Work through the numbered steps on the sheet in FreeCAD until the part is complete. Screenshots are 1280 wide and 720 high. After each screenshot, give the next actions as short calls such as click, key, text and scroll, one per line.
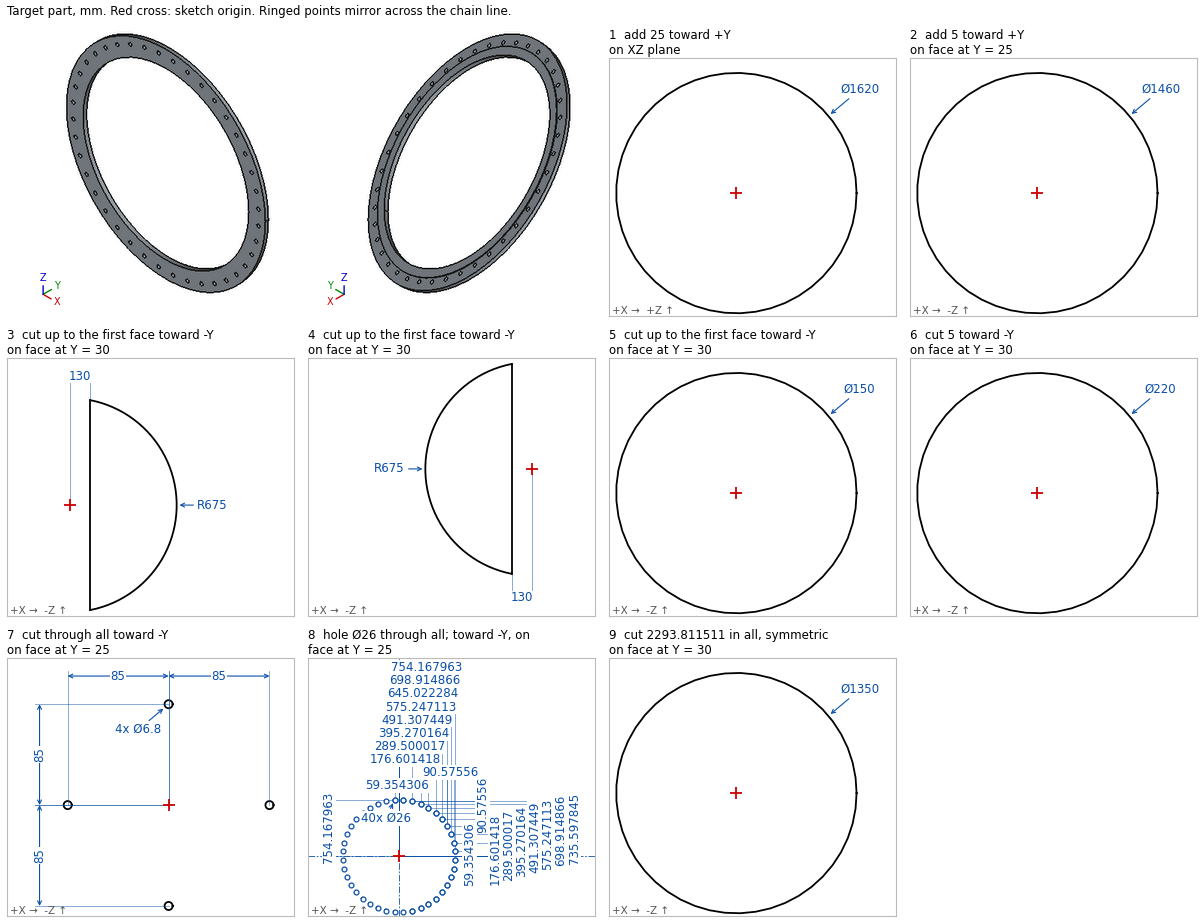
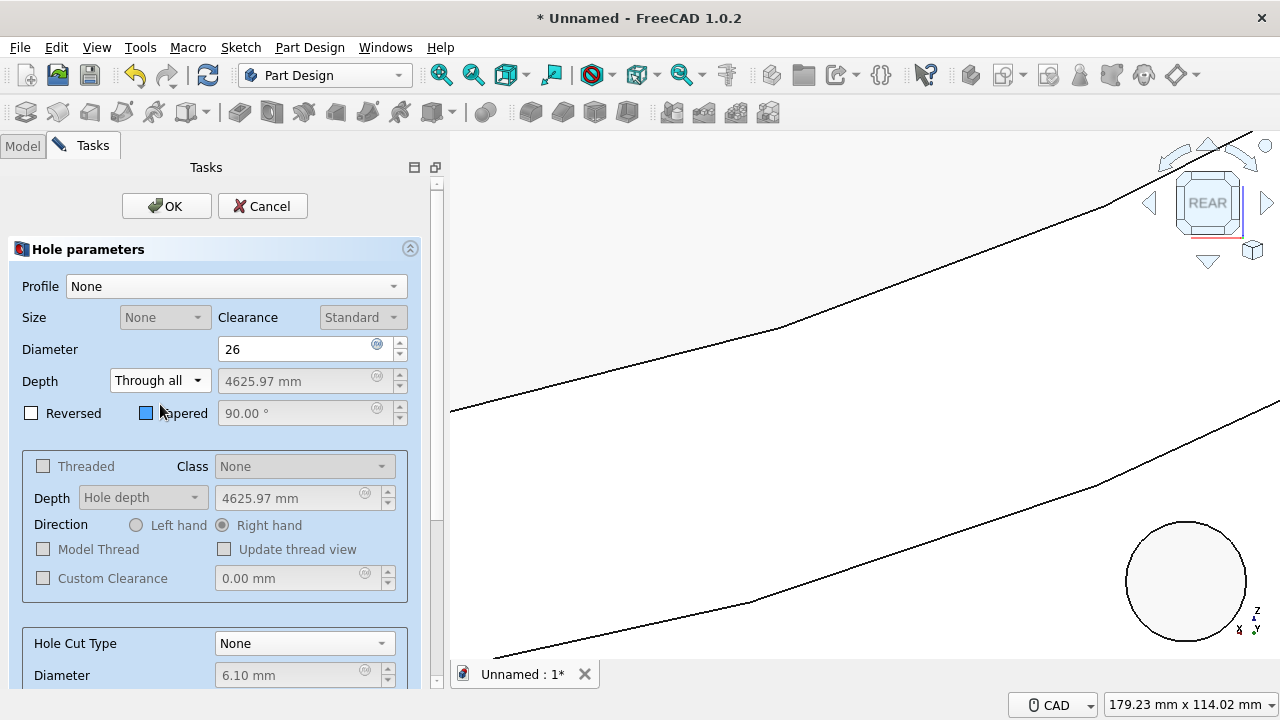
click(167, 206)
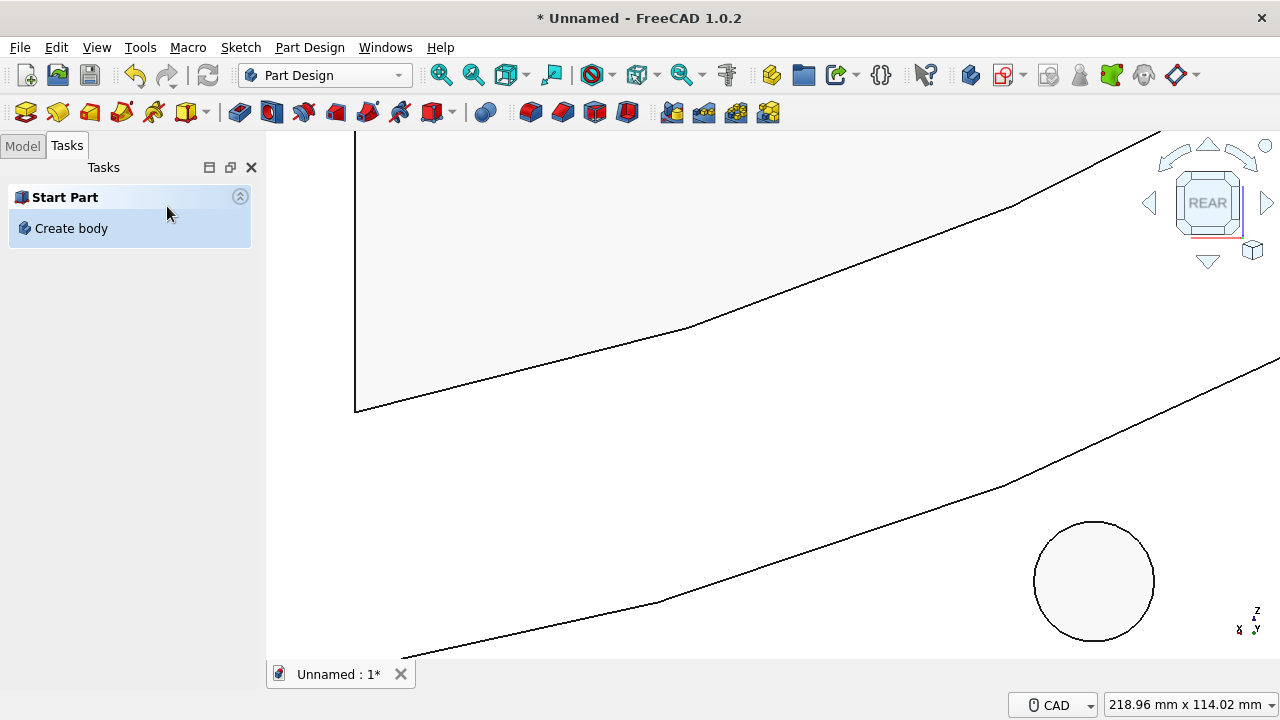
click(442, 76)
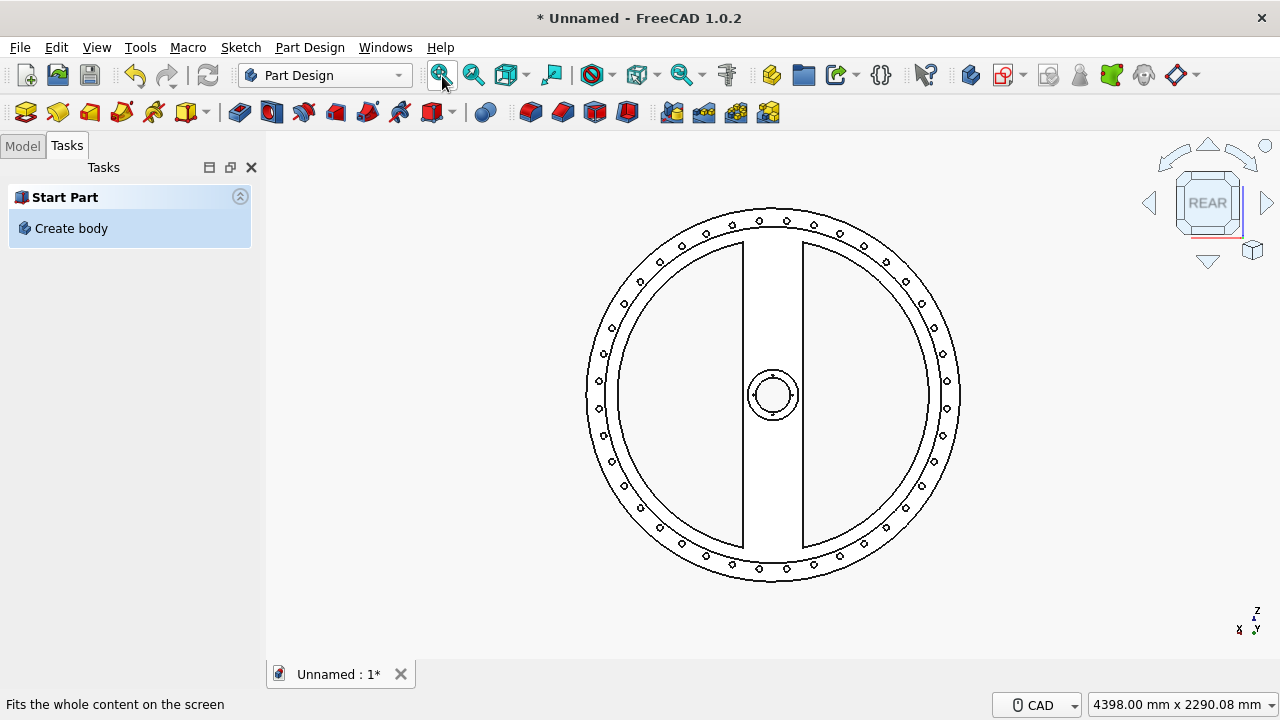
click(773, 490)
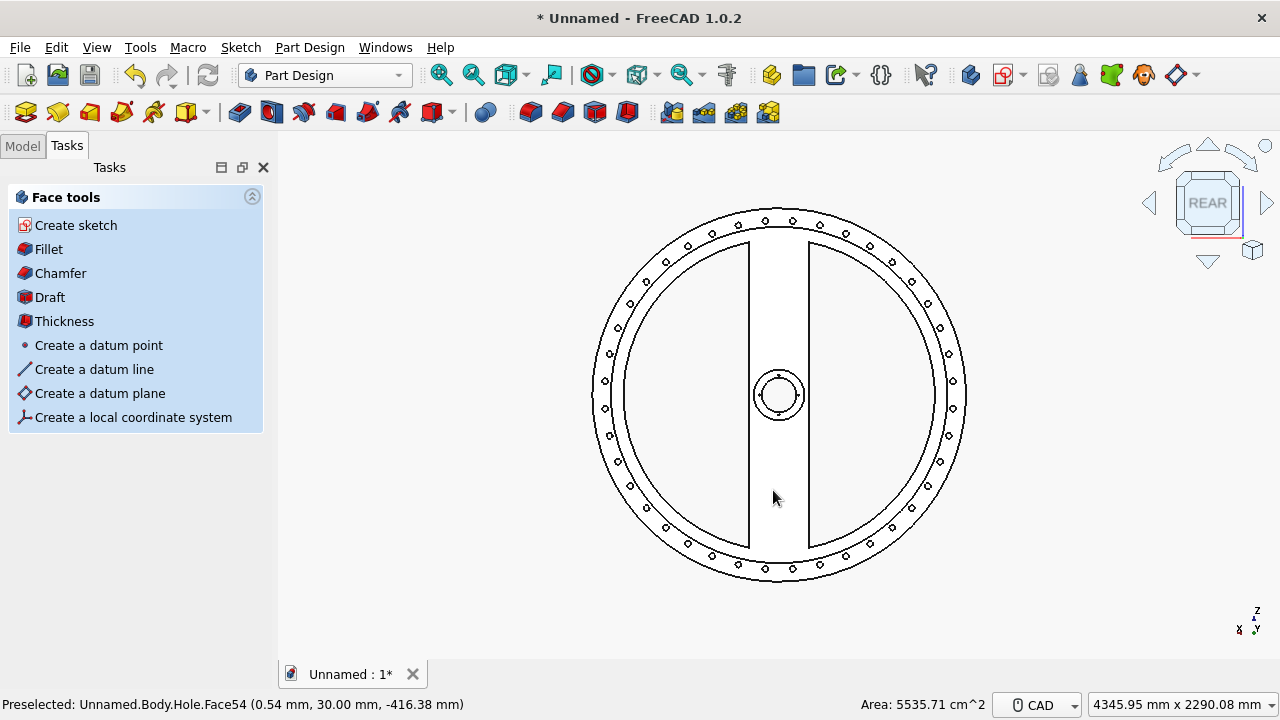
click(1004, 76)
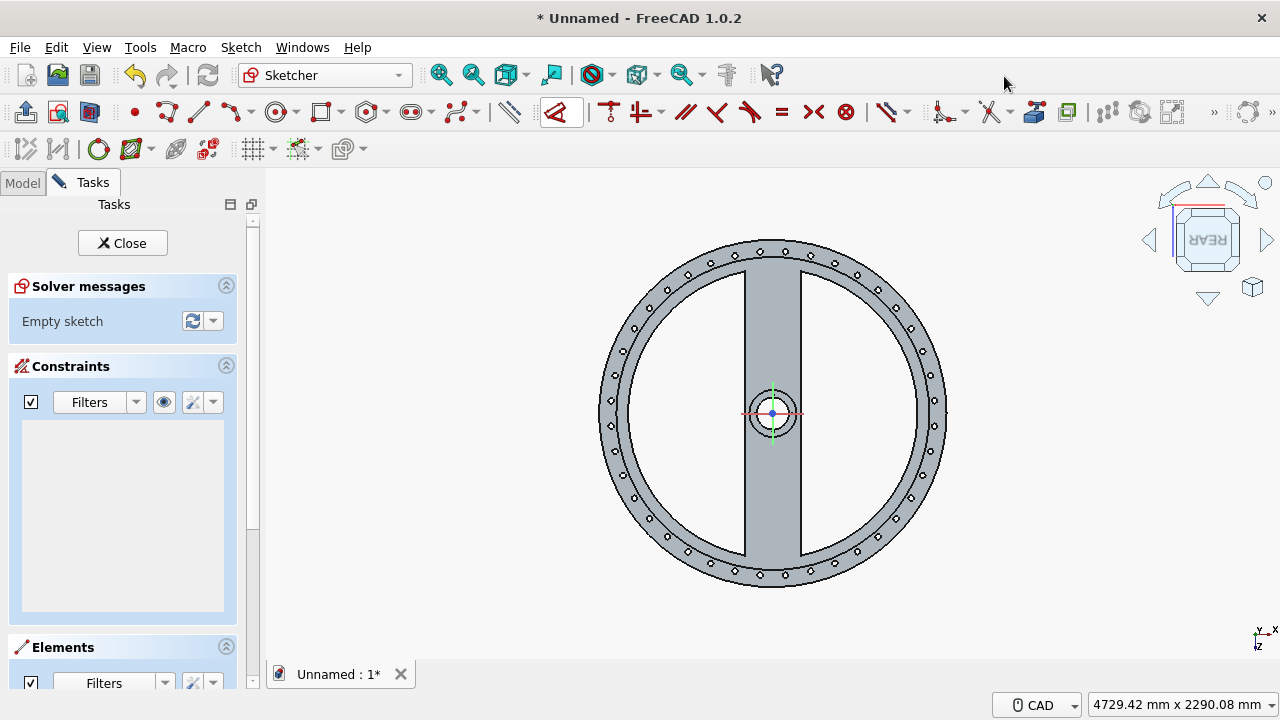
click(276, 112)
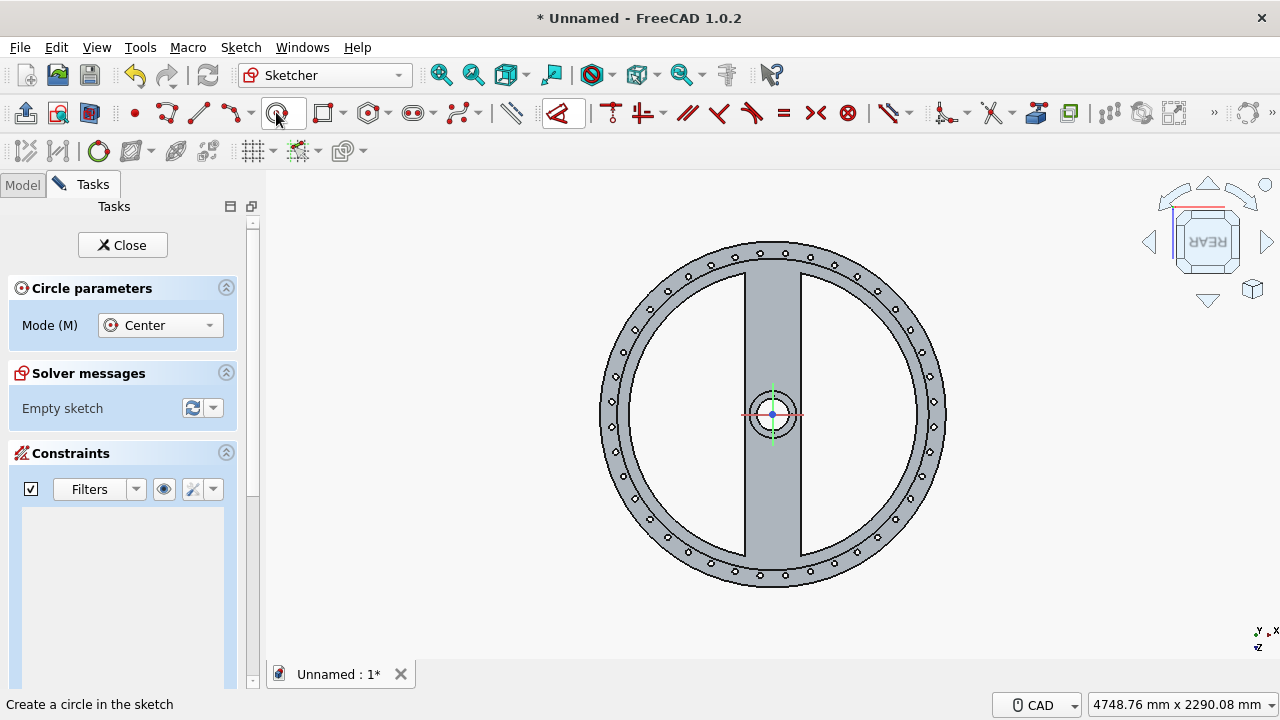
click(773, 414)
click(875, 313)
key(Escape)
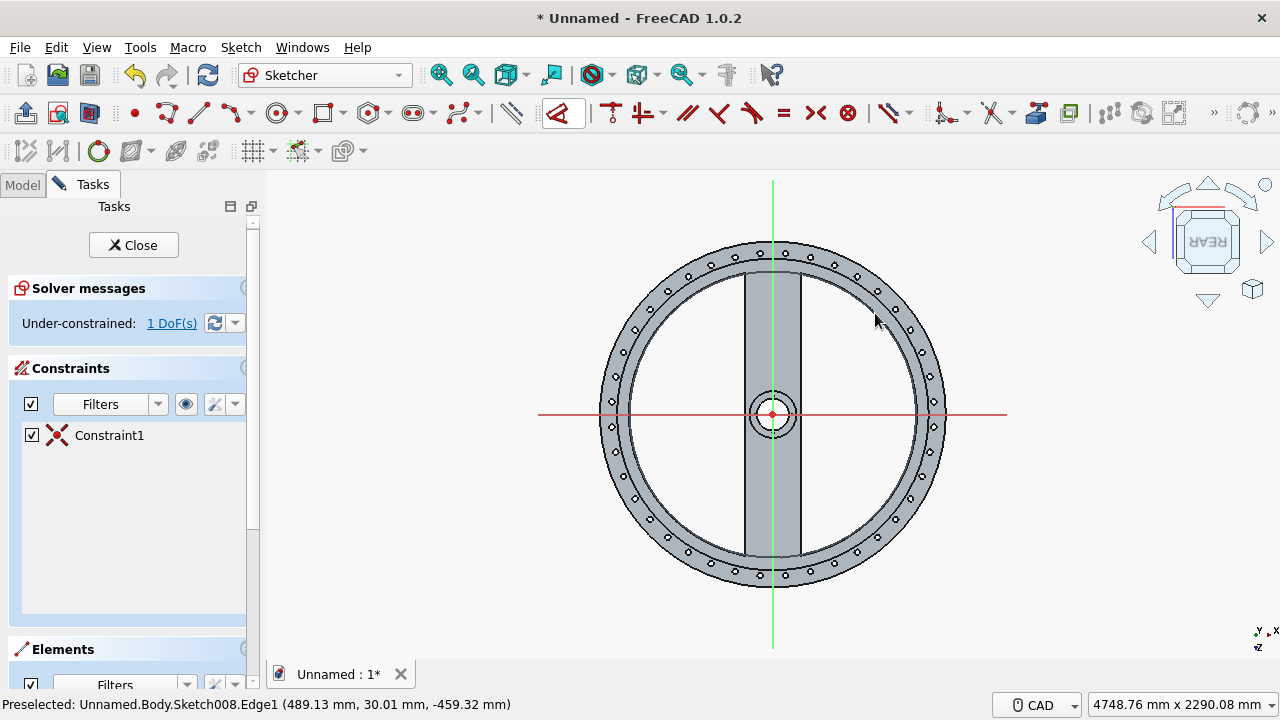
click(874, 313)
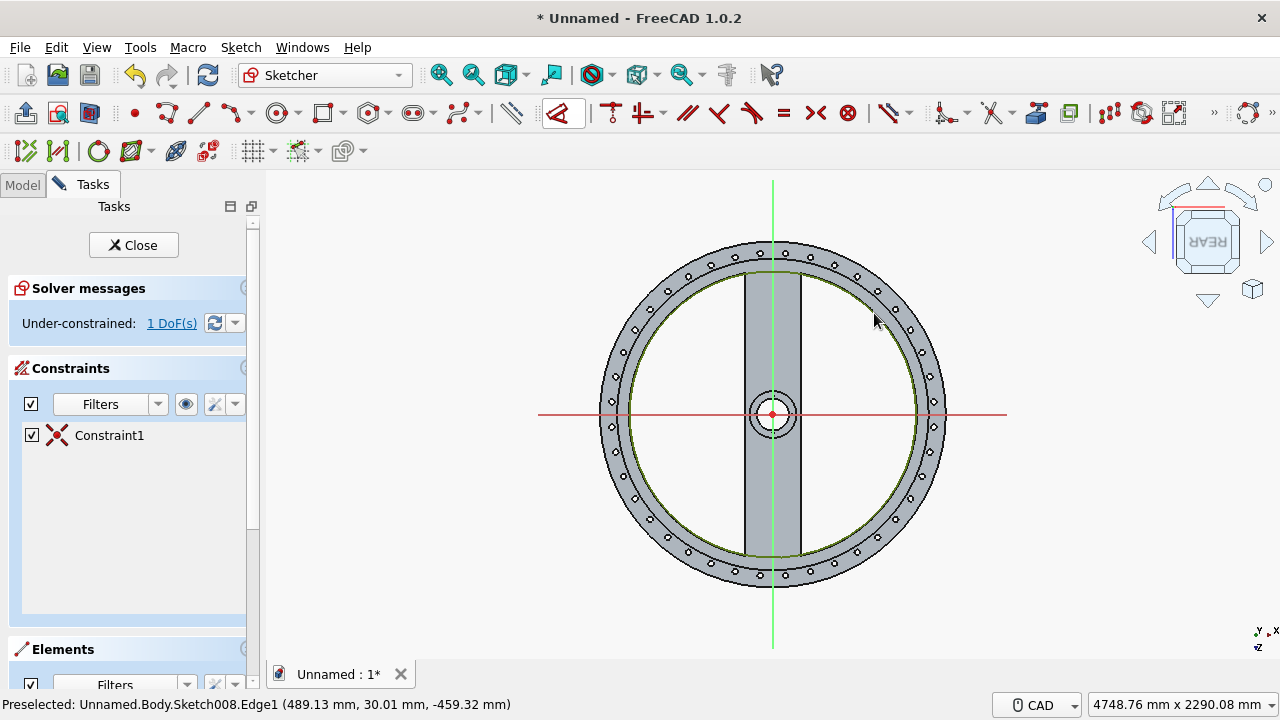
key(k)
key(o)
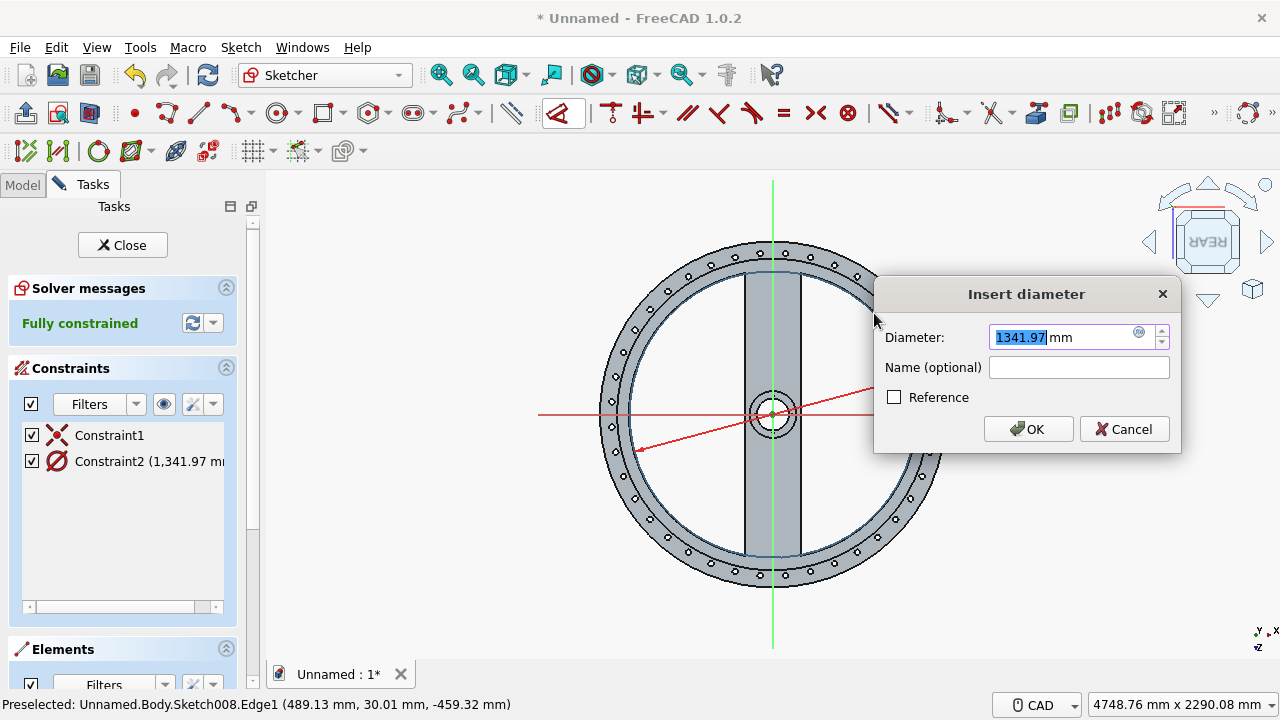
text(1350)
key(Return)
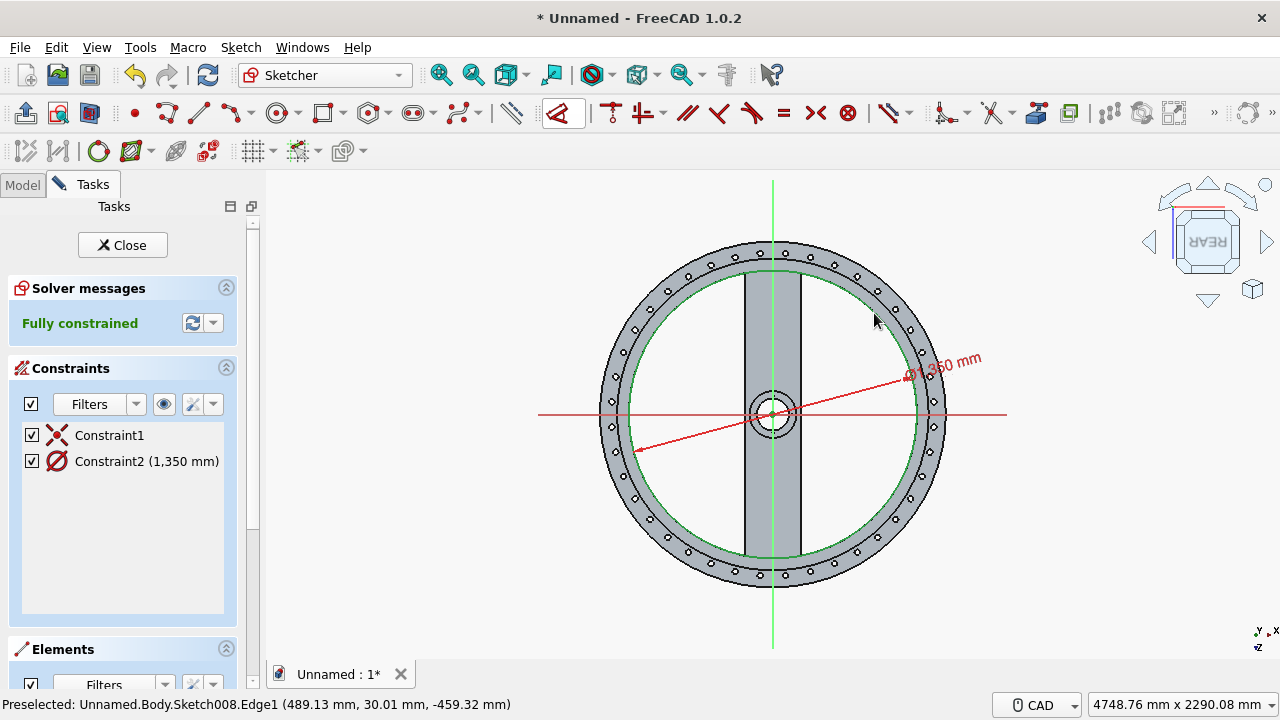
click(123, 245)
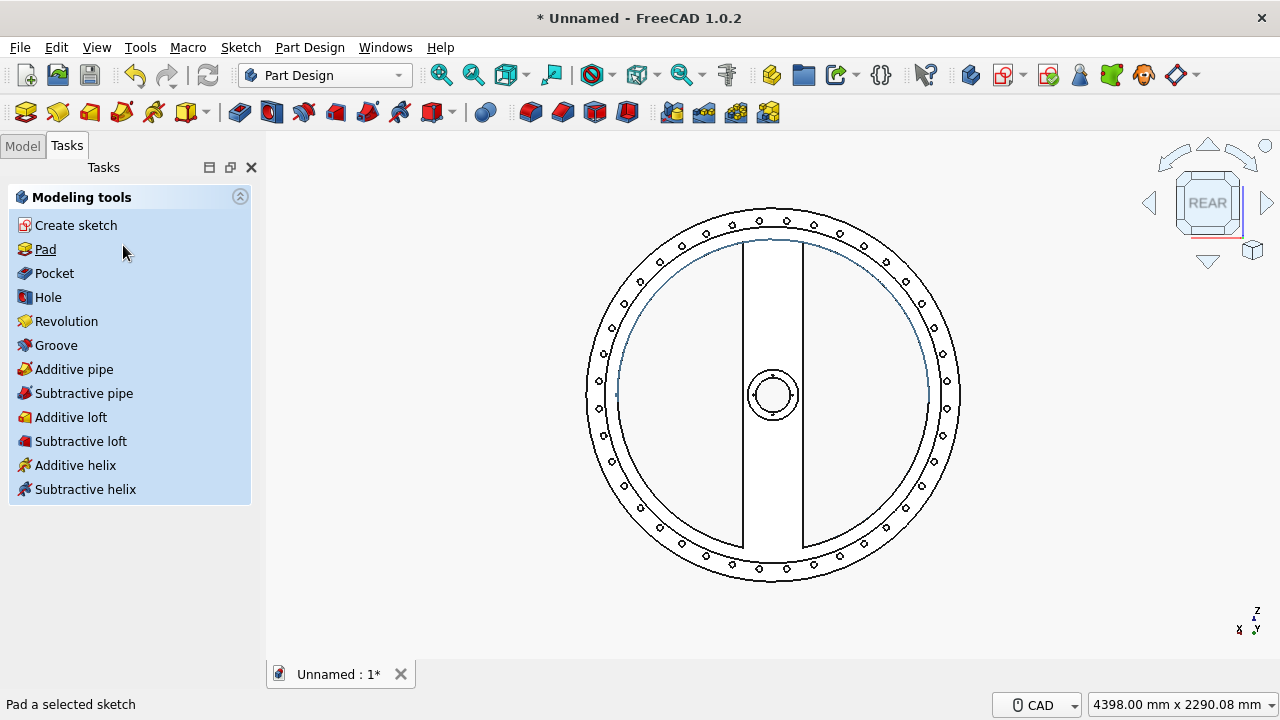
click(240, 112)